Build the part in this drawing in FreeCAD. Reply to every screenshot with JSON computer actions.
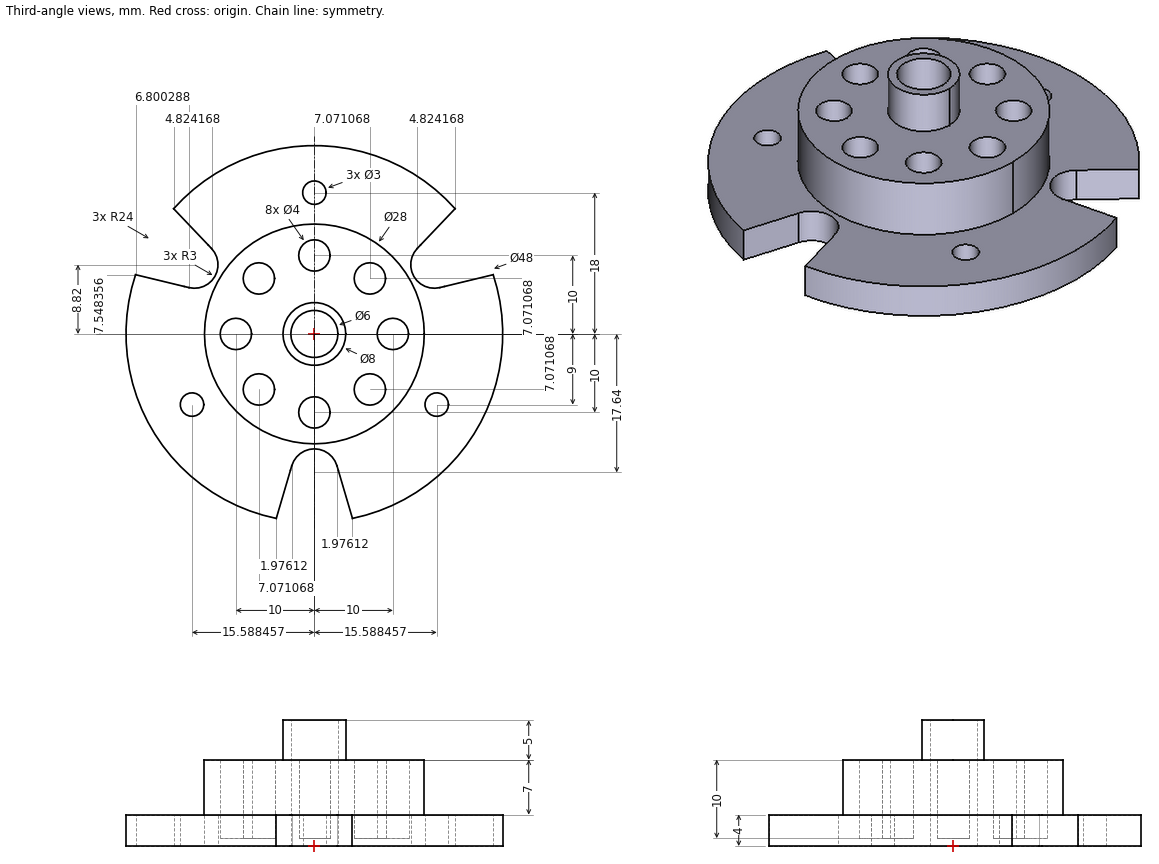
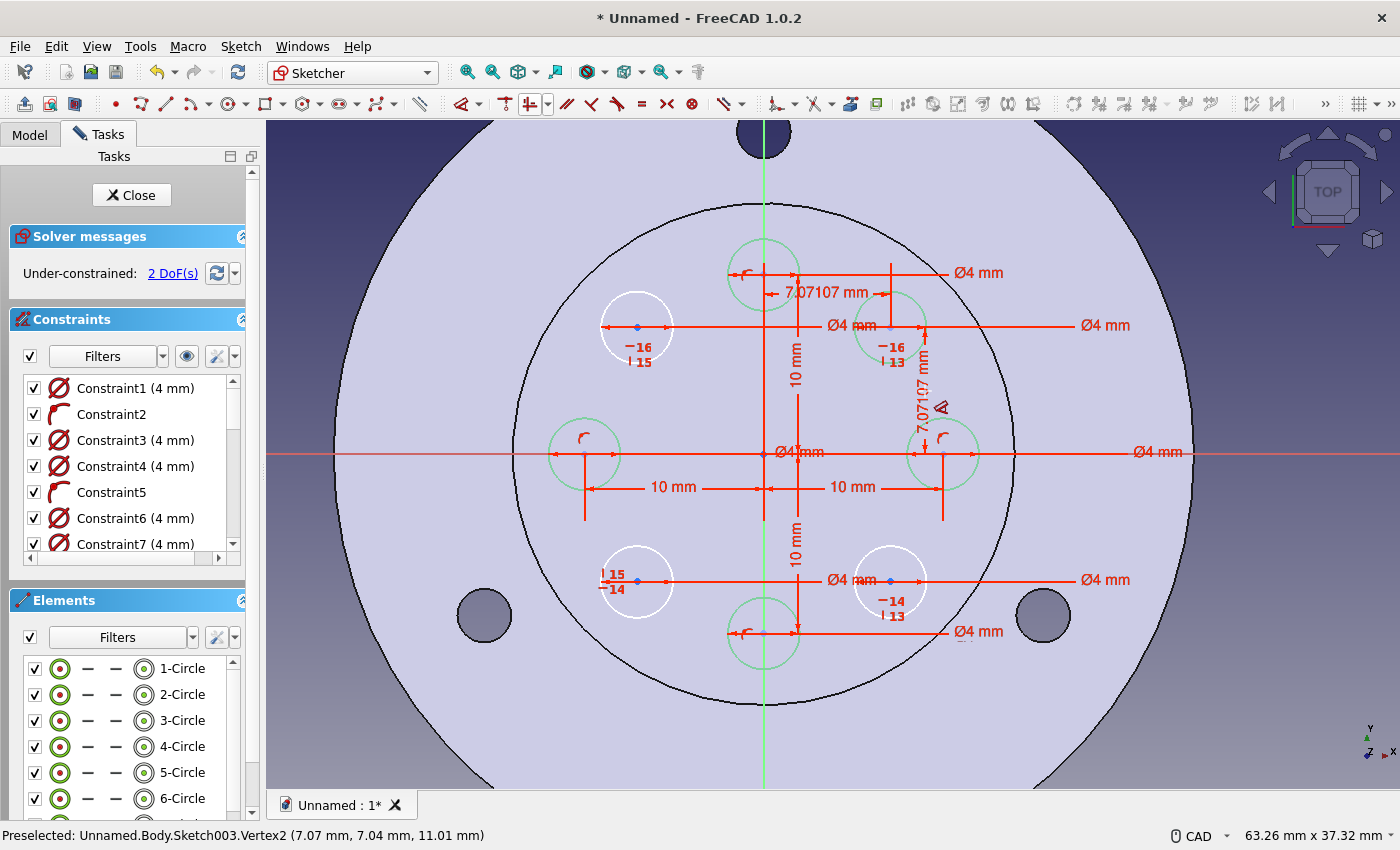
{"action": "left_click", "coordinate": [891, 582]}
{"action": "left_click", "coordinate": [925, 518]}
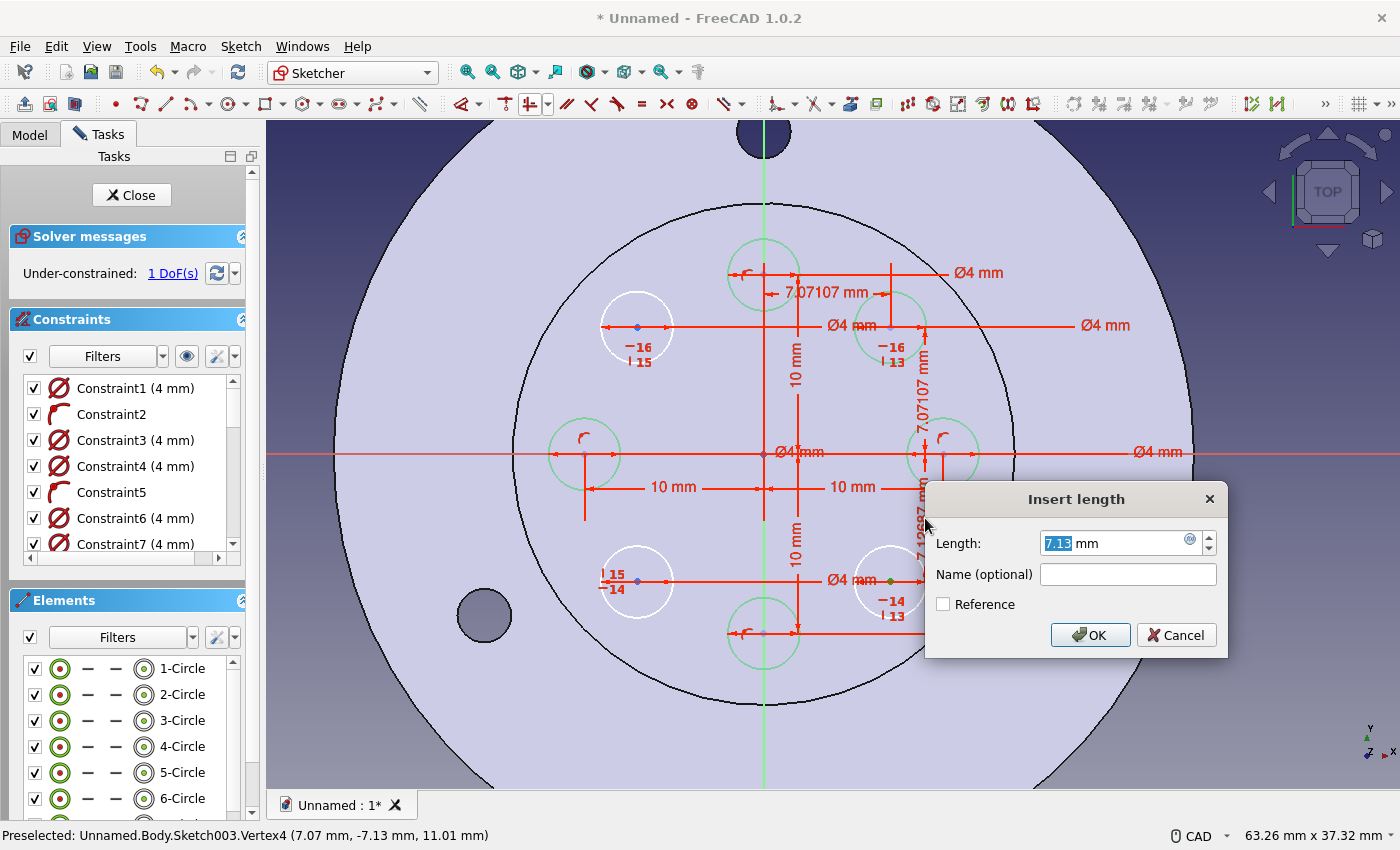
{"action": "type", "text": "7.071068"}
{"action": "key", "text": "Return"}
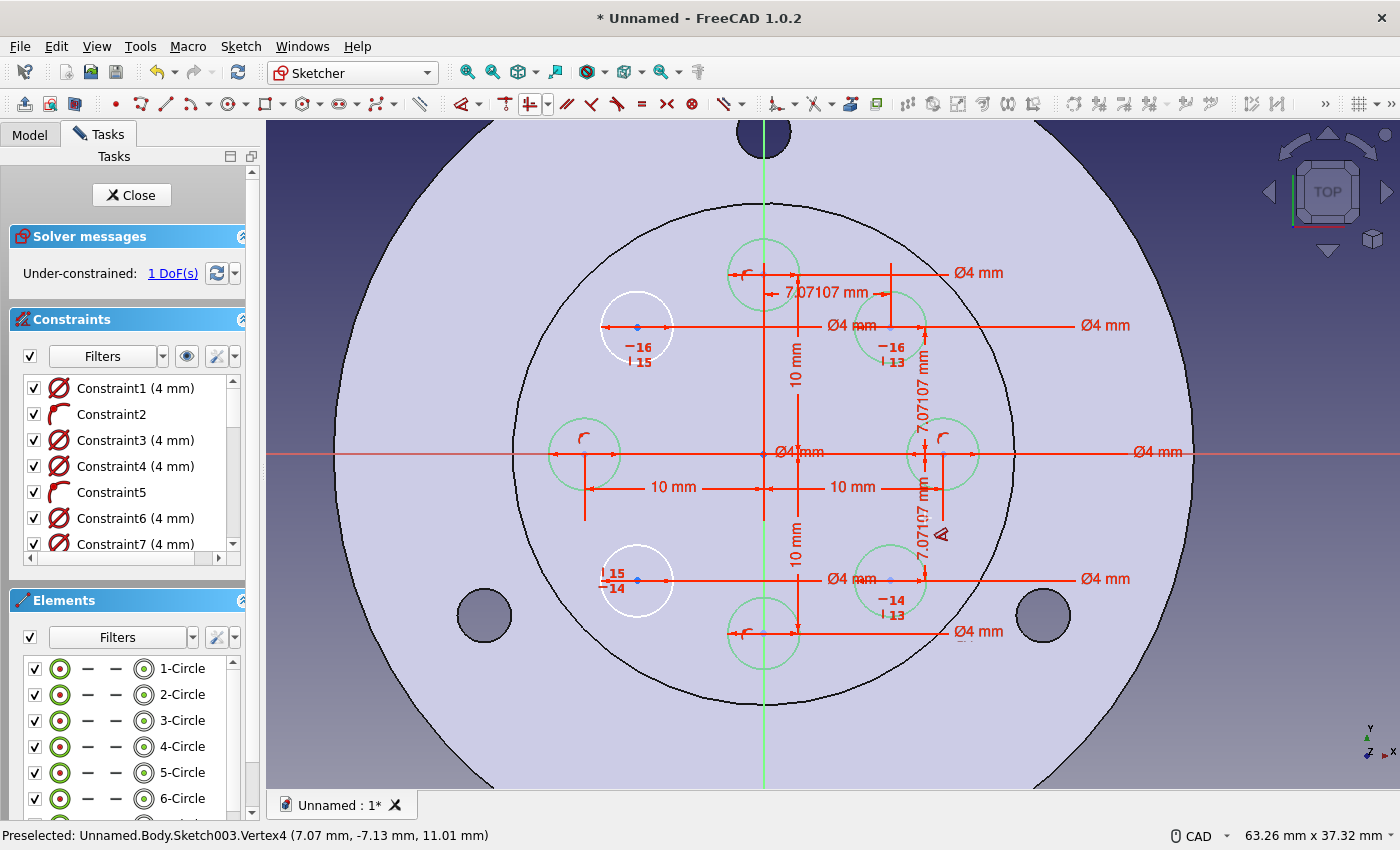
{"action": "left_click", "coordinate": [637, 581]}
{"action": "left_click", "coordinate": [700, 615]}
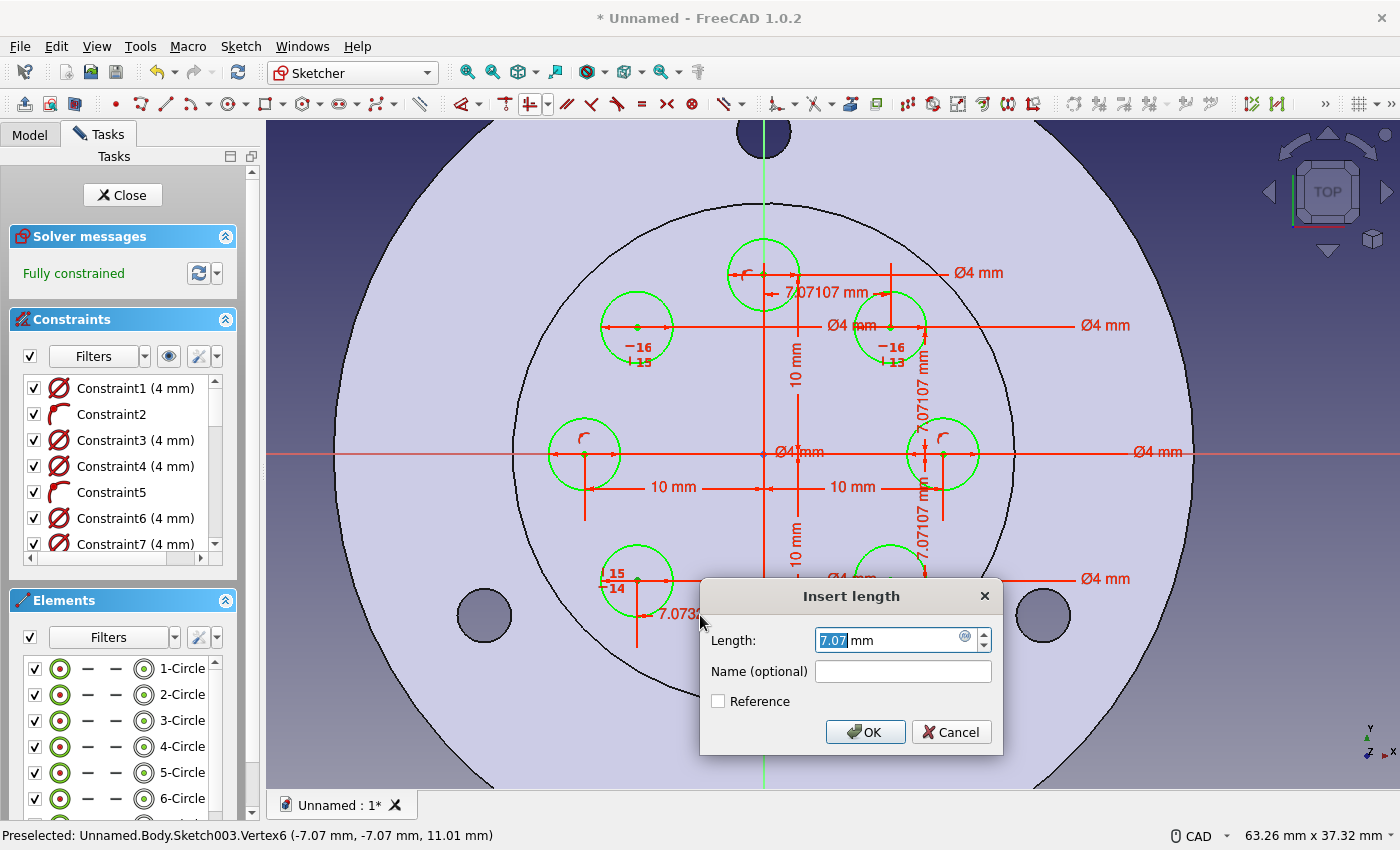
{"action": "type", "text": "7.071068"}
{"action": "key", "text": "Return"}
{"action": "key", "text": "Escape"}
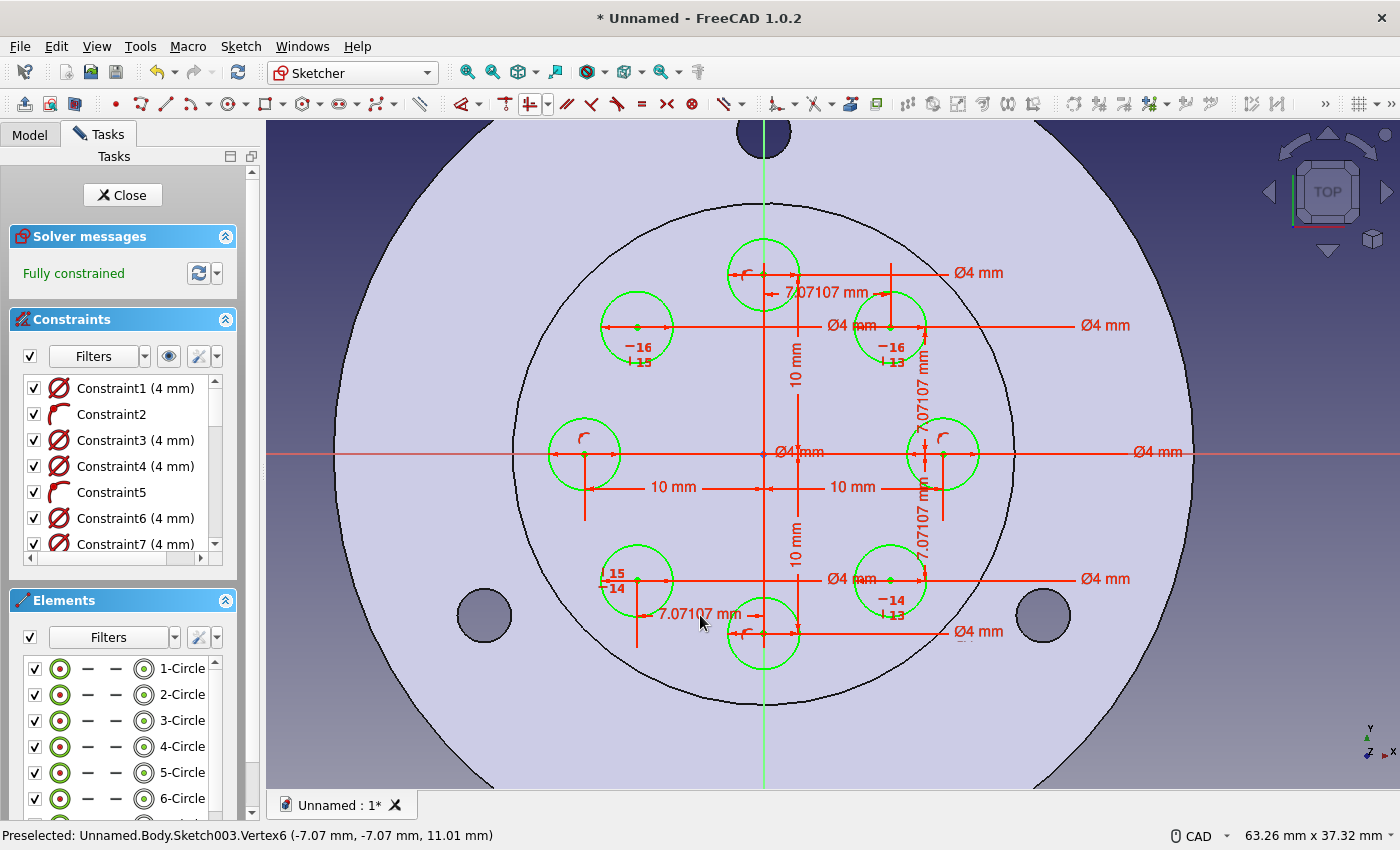
{"action": "left_click", "coordinate": [123, 195]}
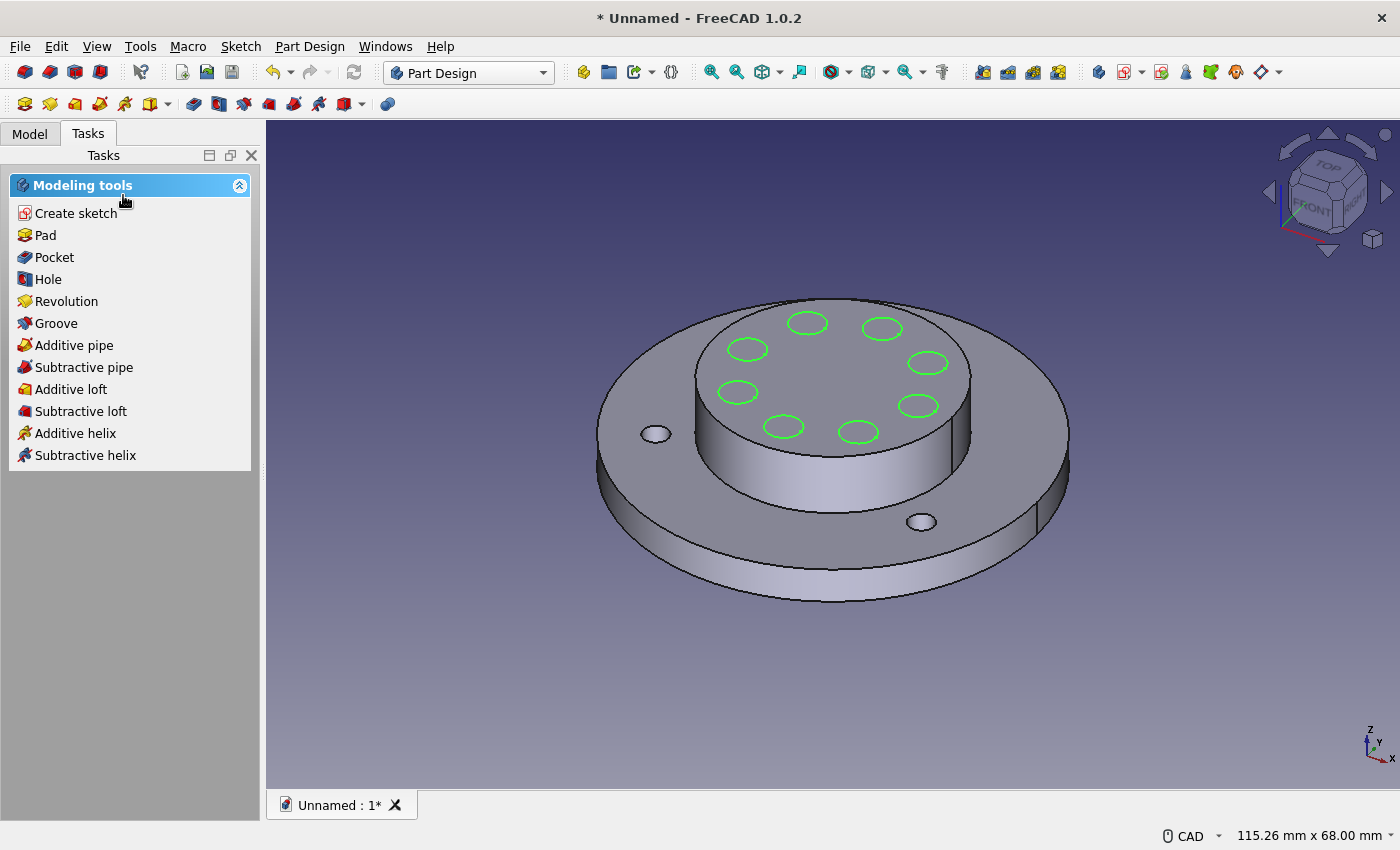
{"action": "left_click", "coordinate": [194, 104]}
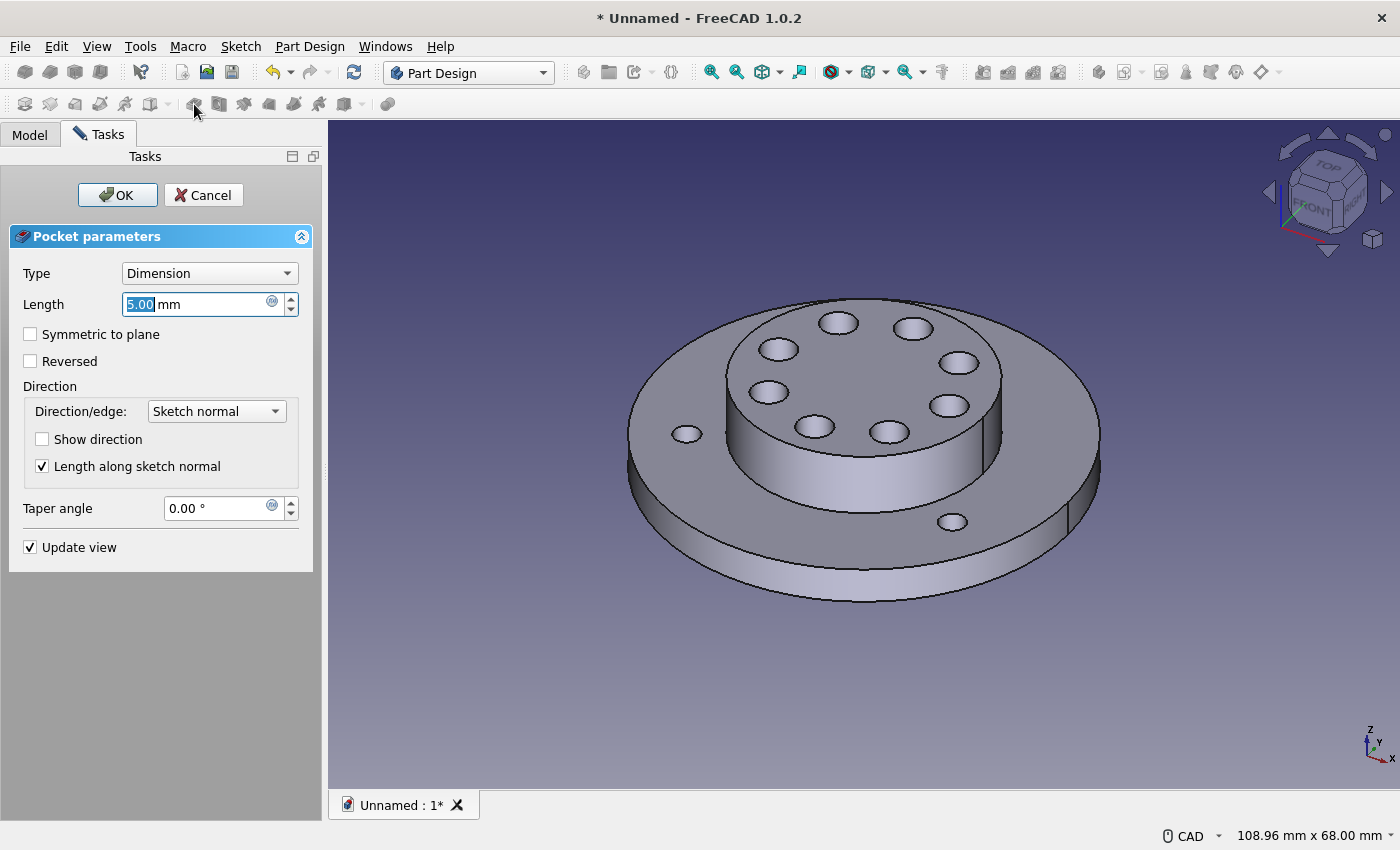
{"action": "type", "text": "10"}
{"action": "key", "text": "Tab"}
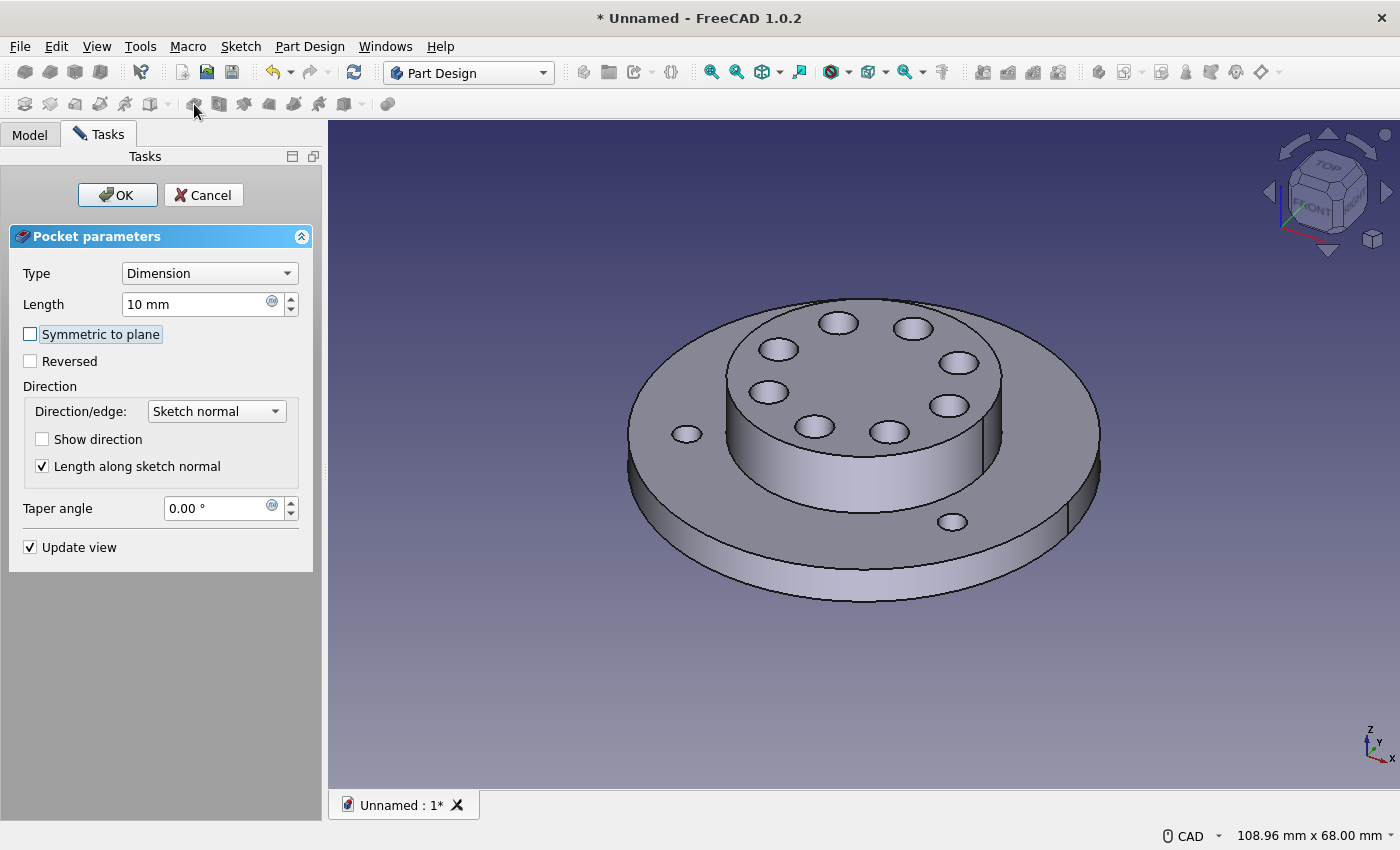
{"action": "left_click", "coordinate": [118, 195]}